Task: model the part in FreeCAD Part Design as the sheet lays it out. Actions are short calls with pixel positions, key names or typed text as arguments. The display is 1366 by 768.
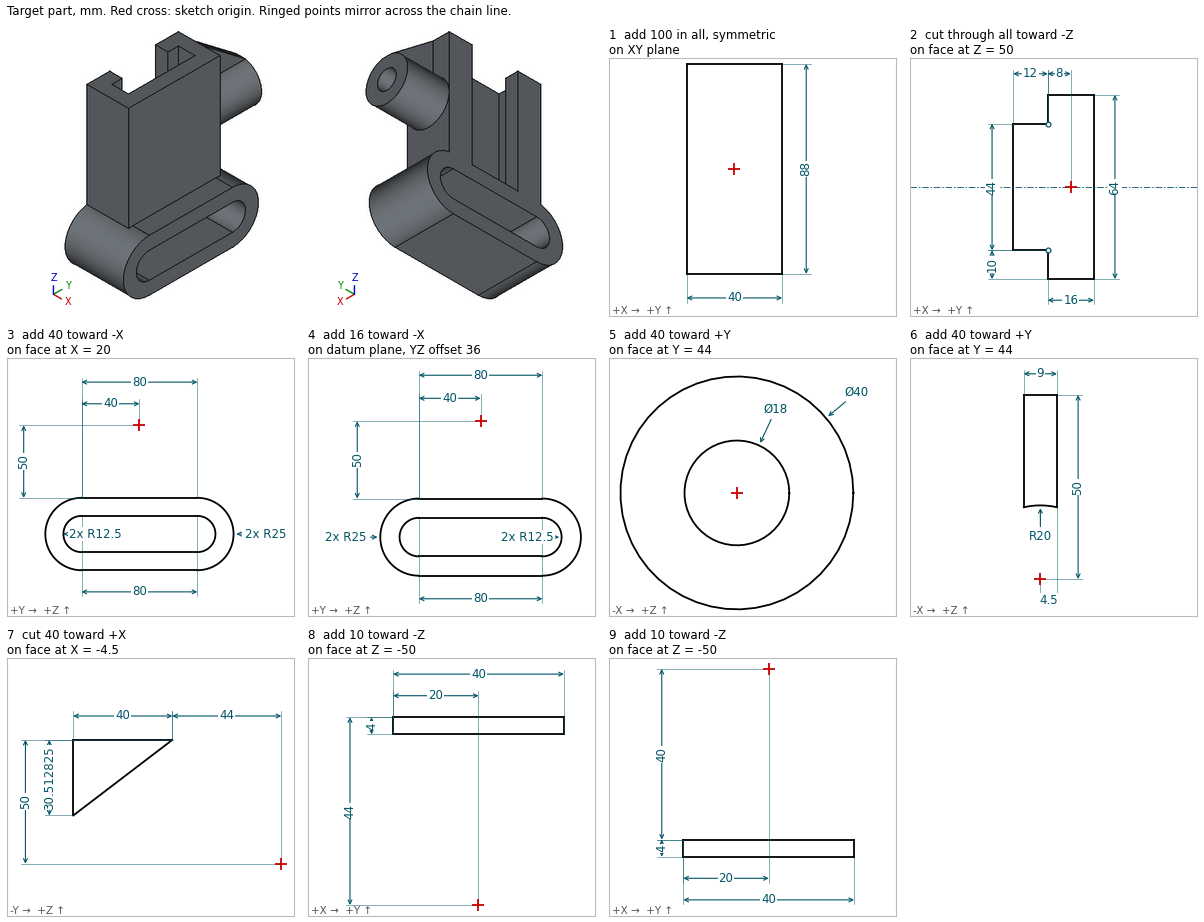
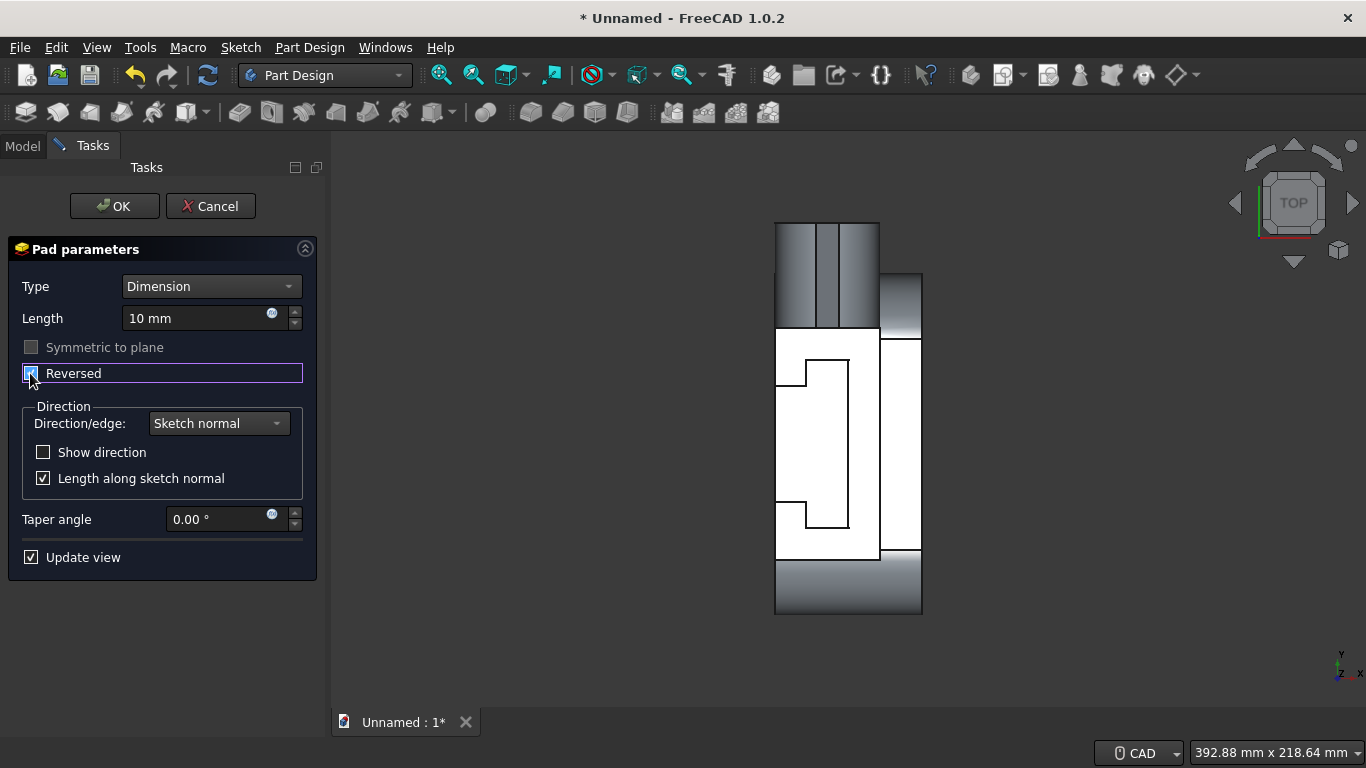
click(115, 206)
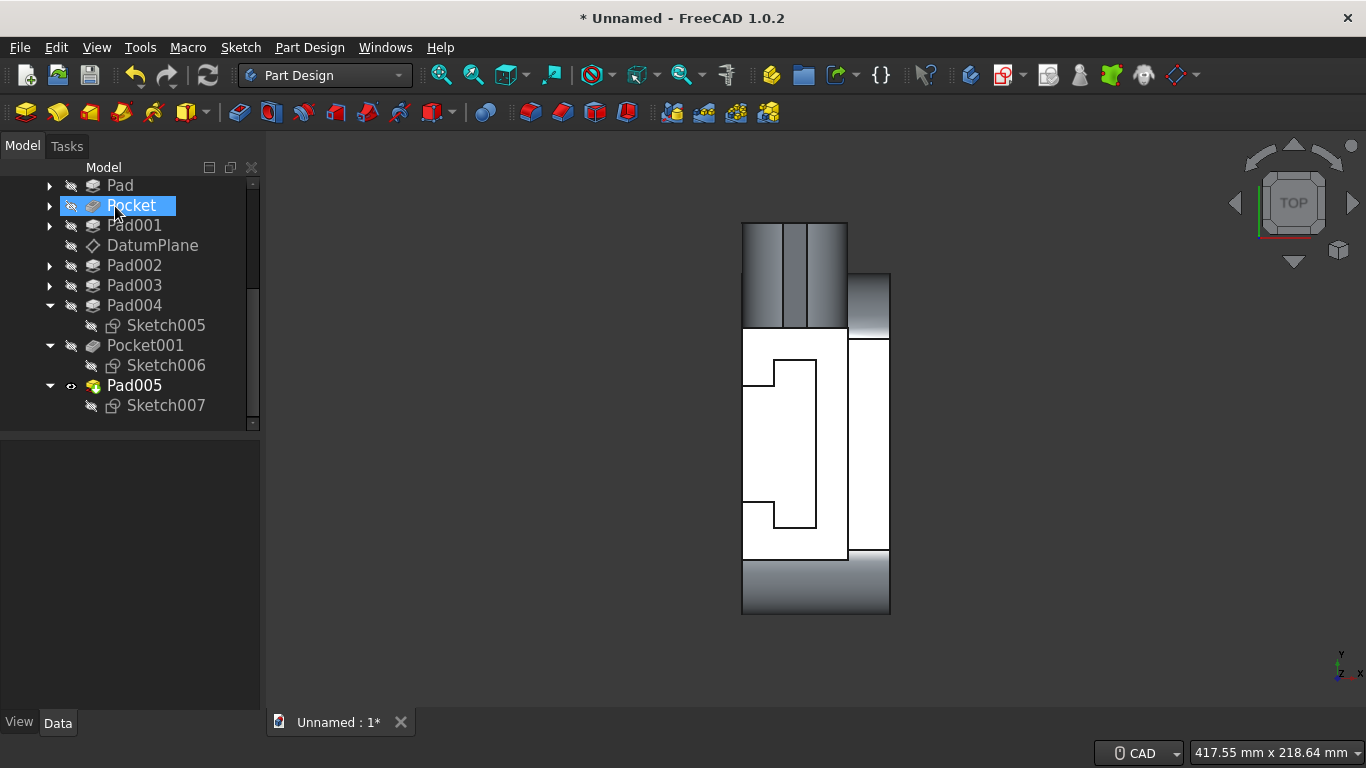
click(779, 443)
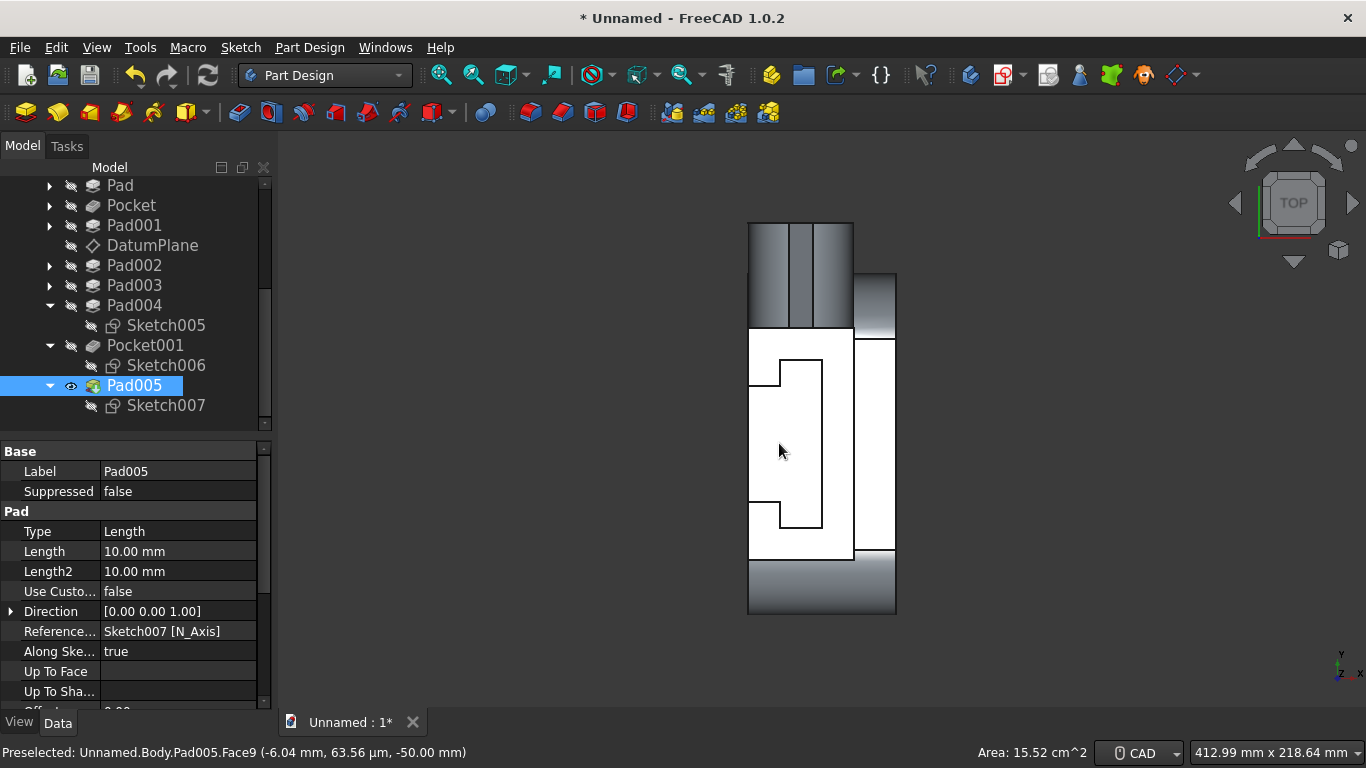
click(1004, 76)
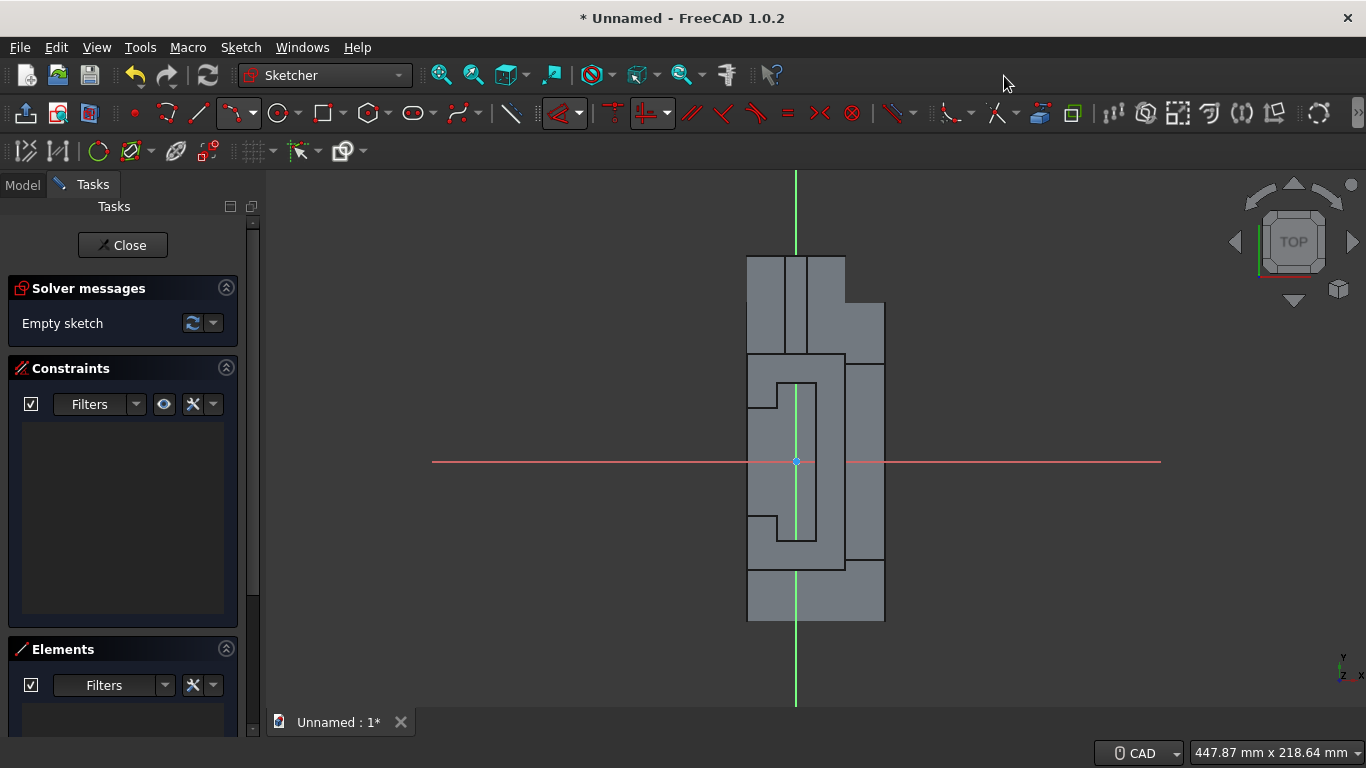
scroll(817, 549, up, 6)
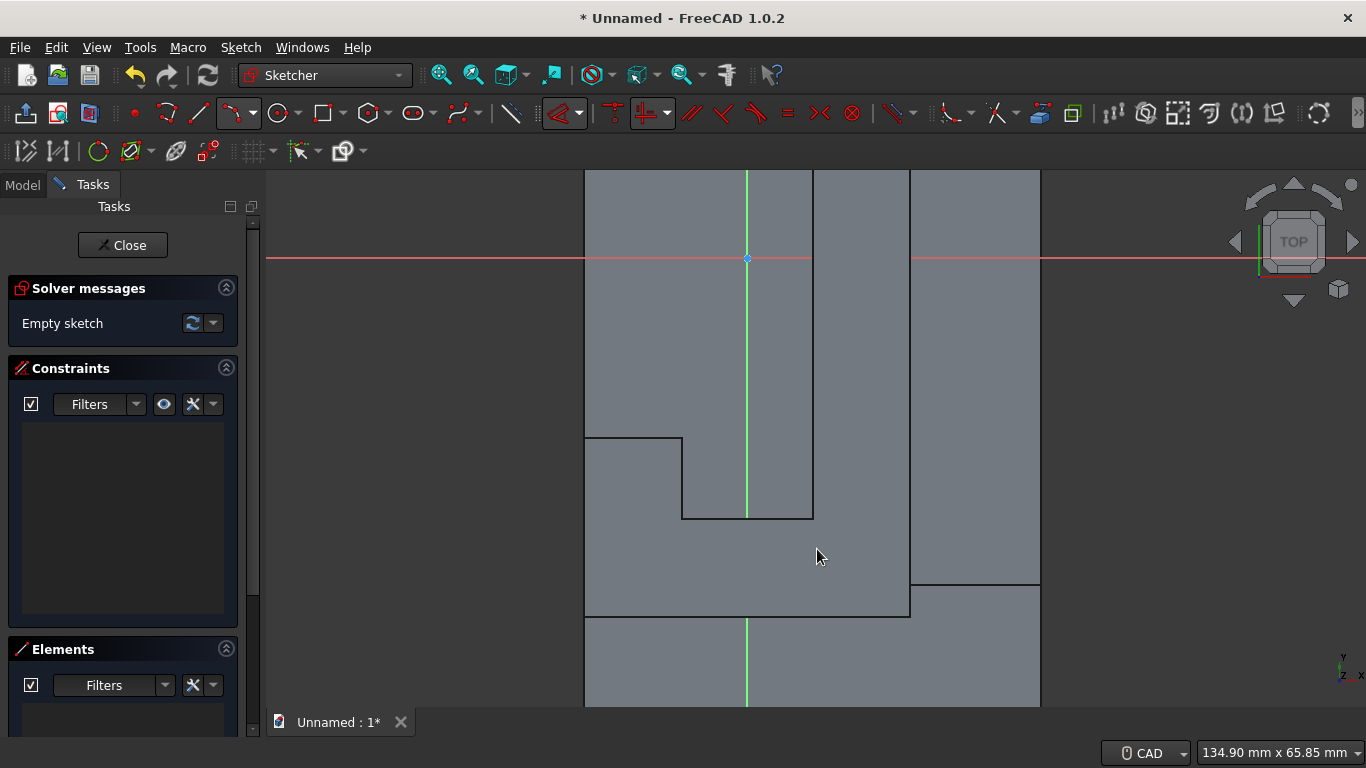
key(g)
key(r)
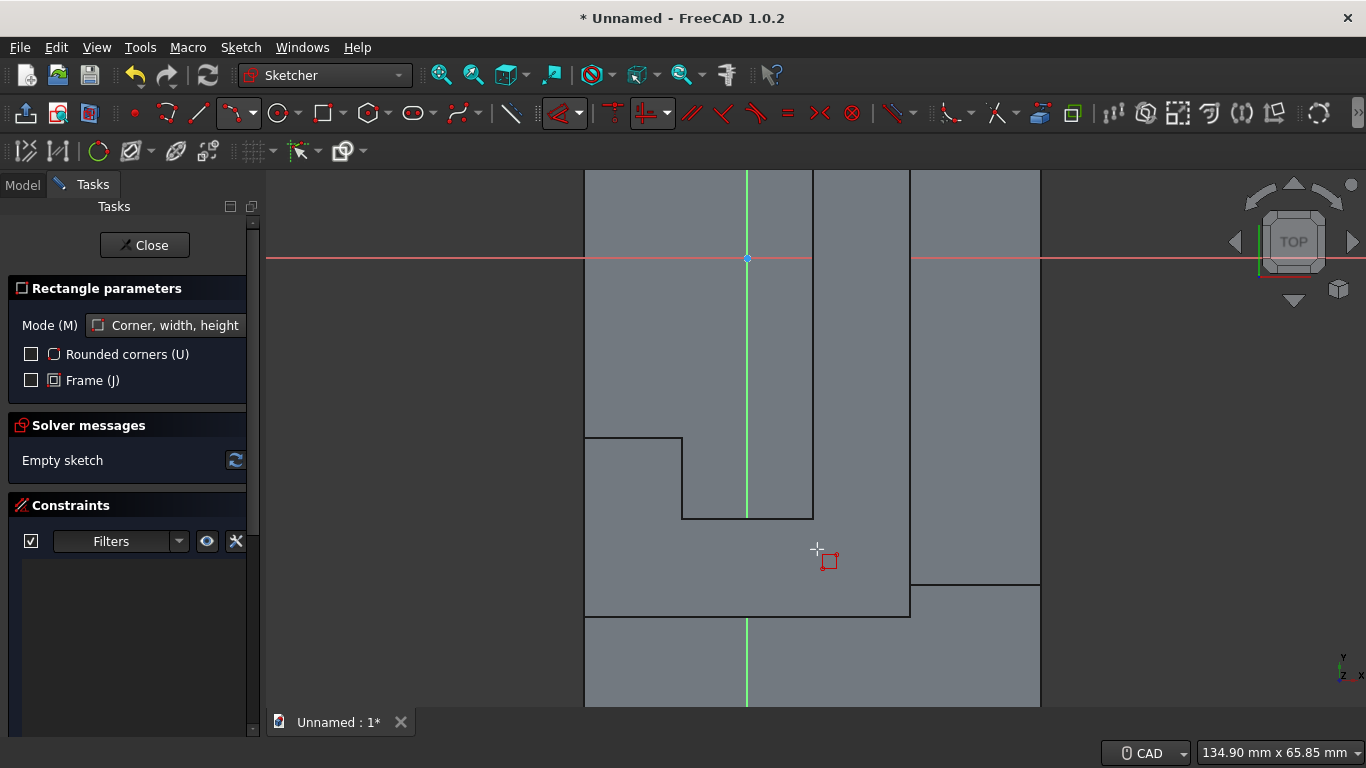
click(584, 585)
click(910, 617)
key(Escape)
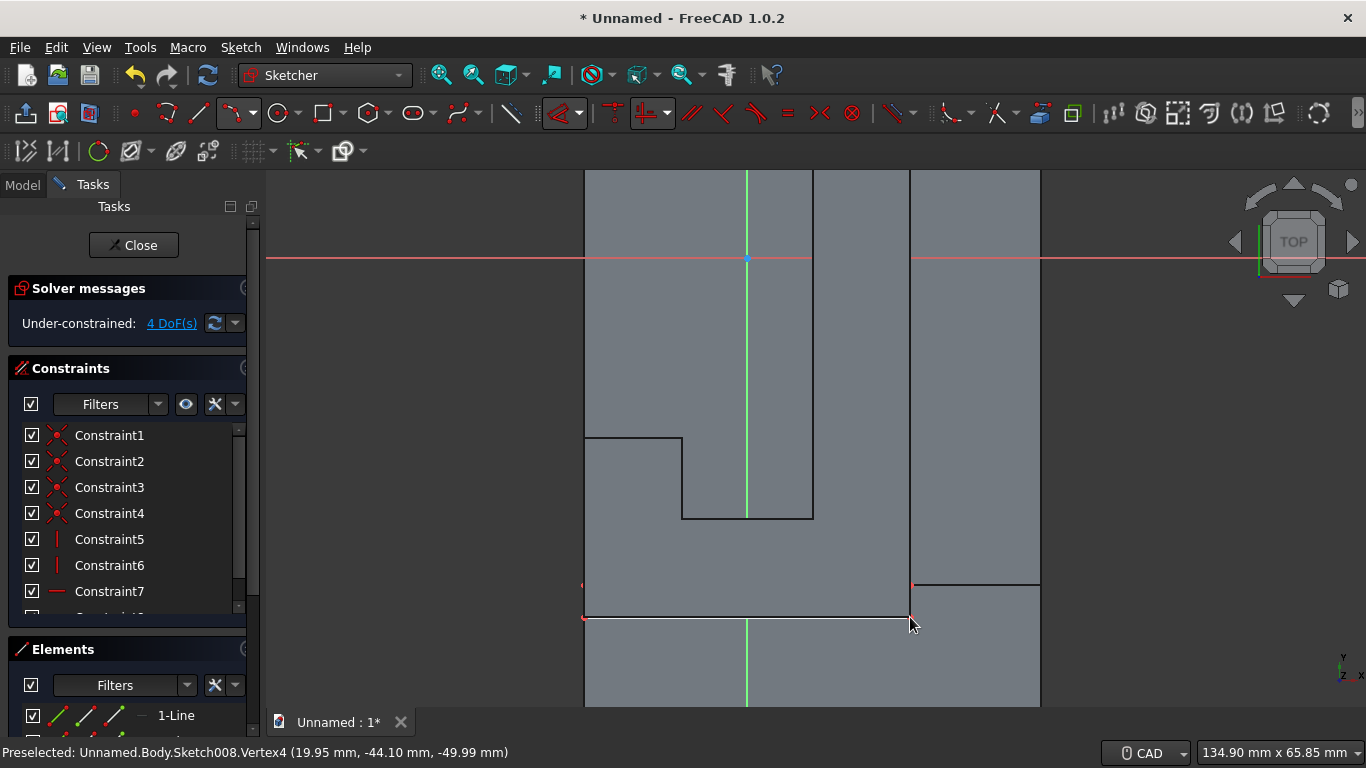
scroll(584, 596, up, 2)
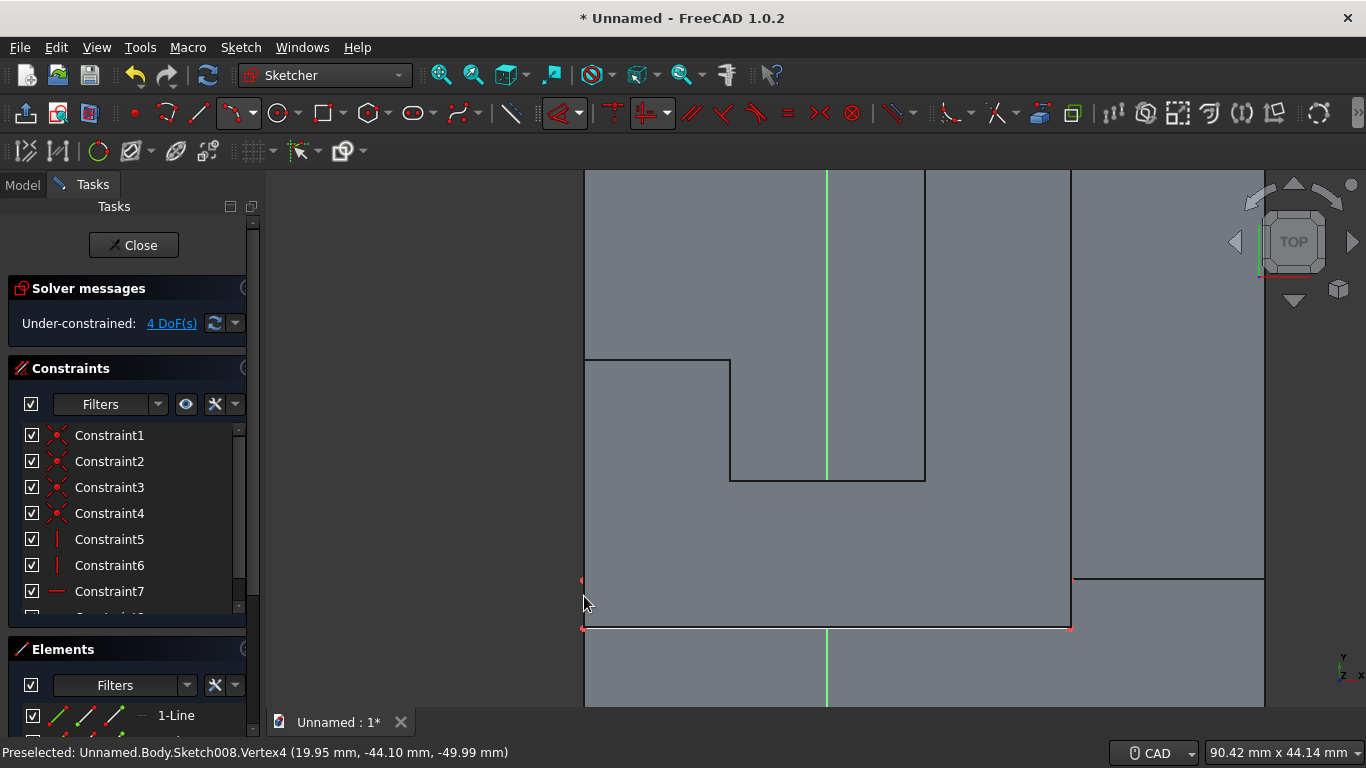
click(584, 595)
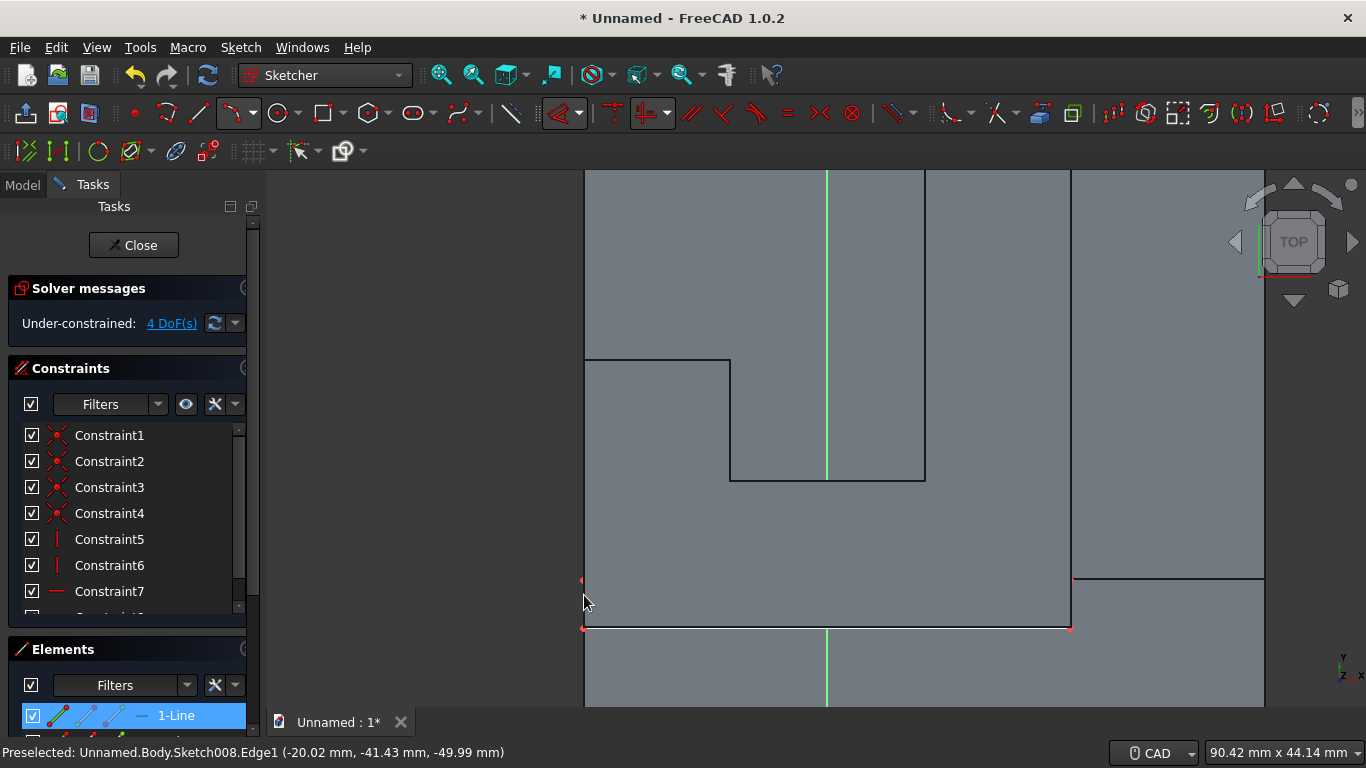
key(i)